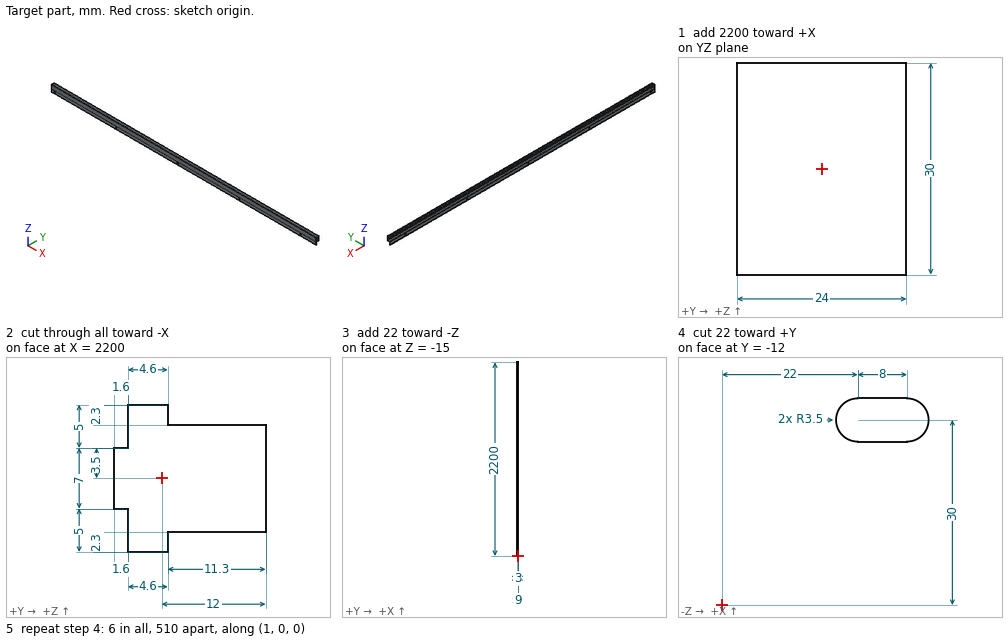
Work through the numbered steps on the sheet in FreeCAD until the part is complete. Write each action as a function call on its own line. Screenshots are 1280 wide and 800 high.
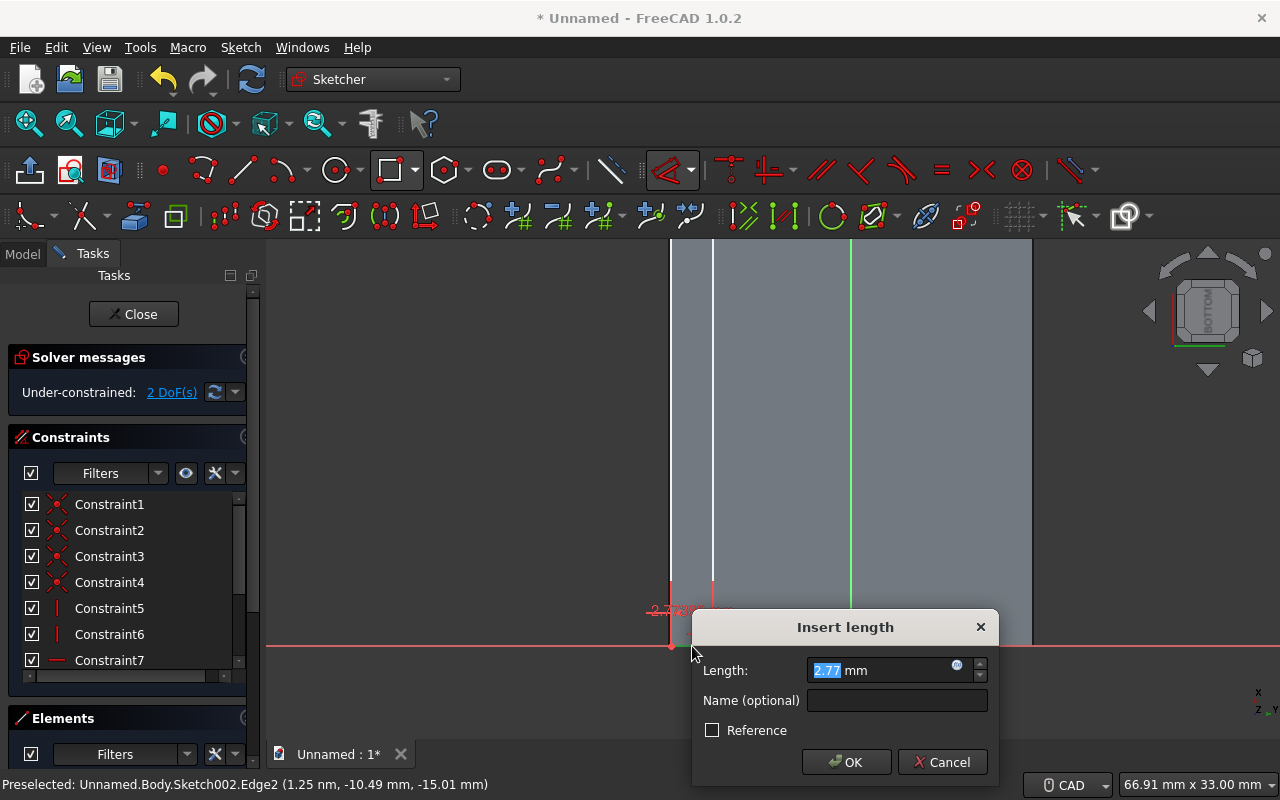
text(3)
key(Return)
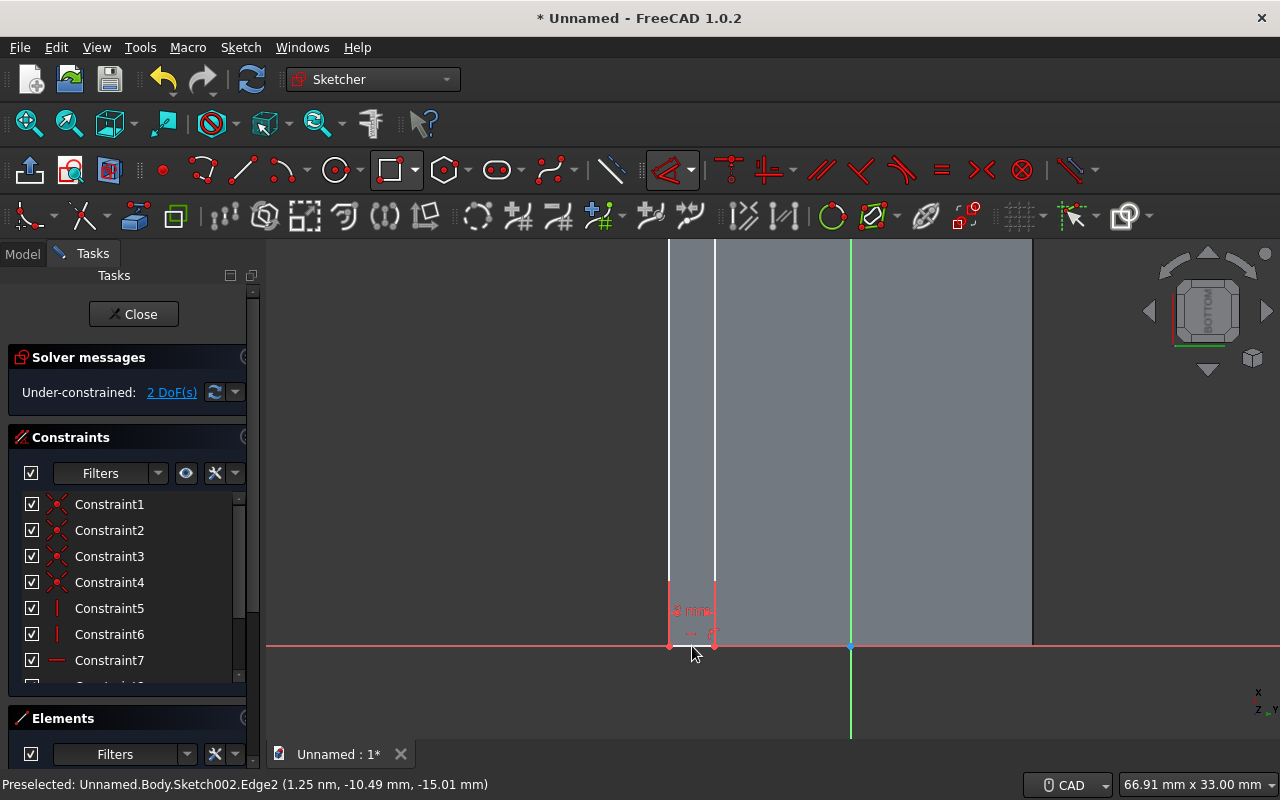
scroll(704, 489, down, 15)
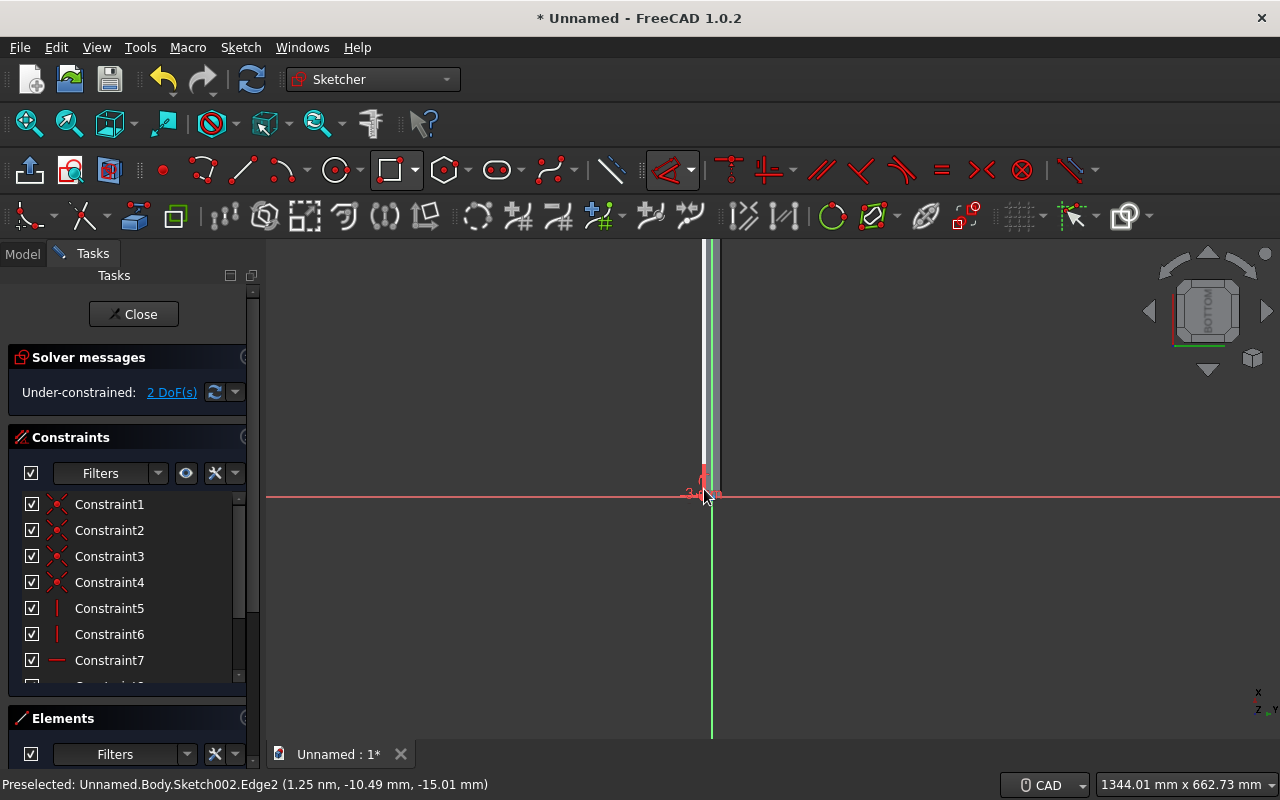
scroll(704, 697, down, 8)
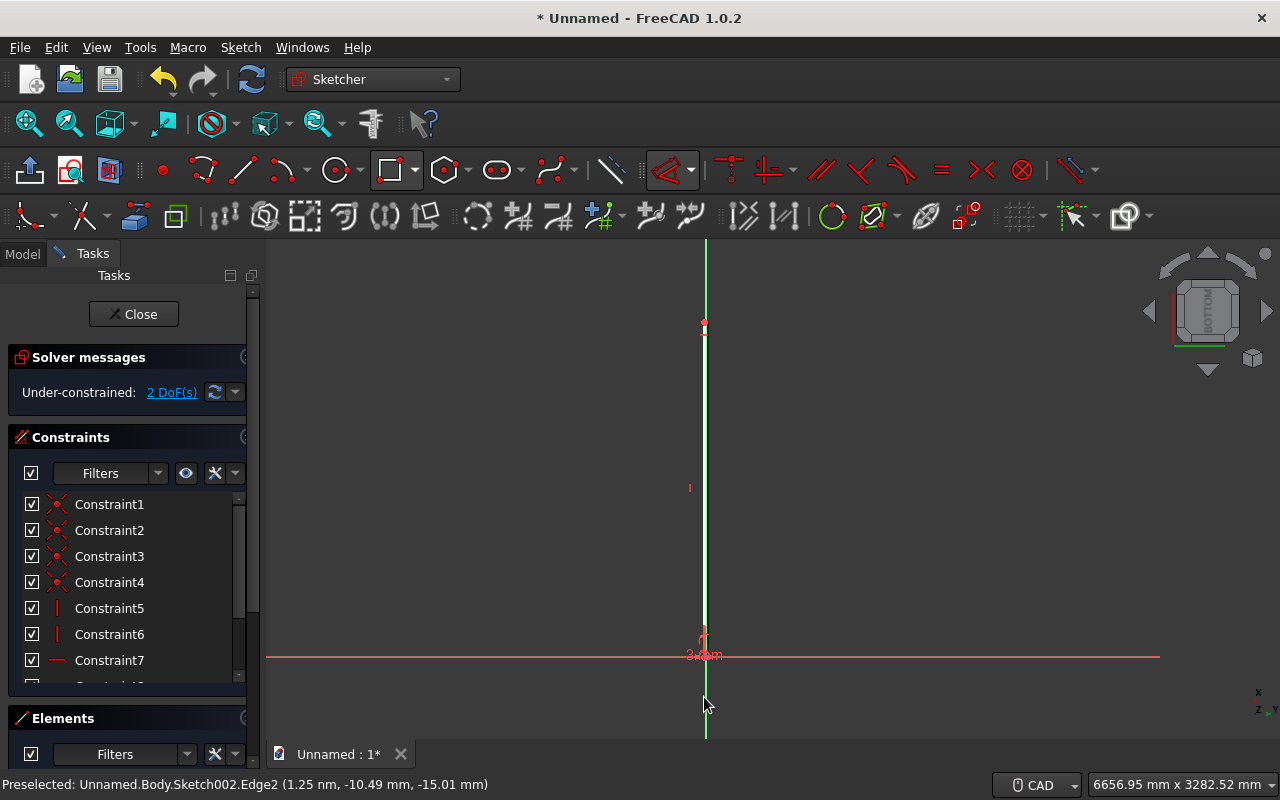
scroll(705, 657, up, 17)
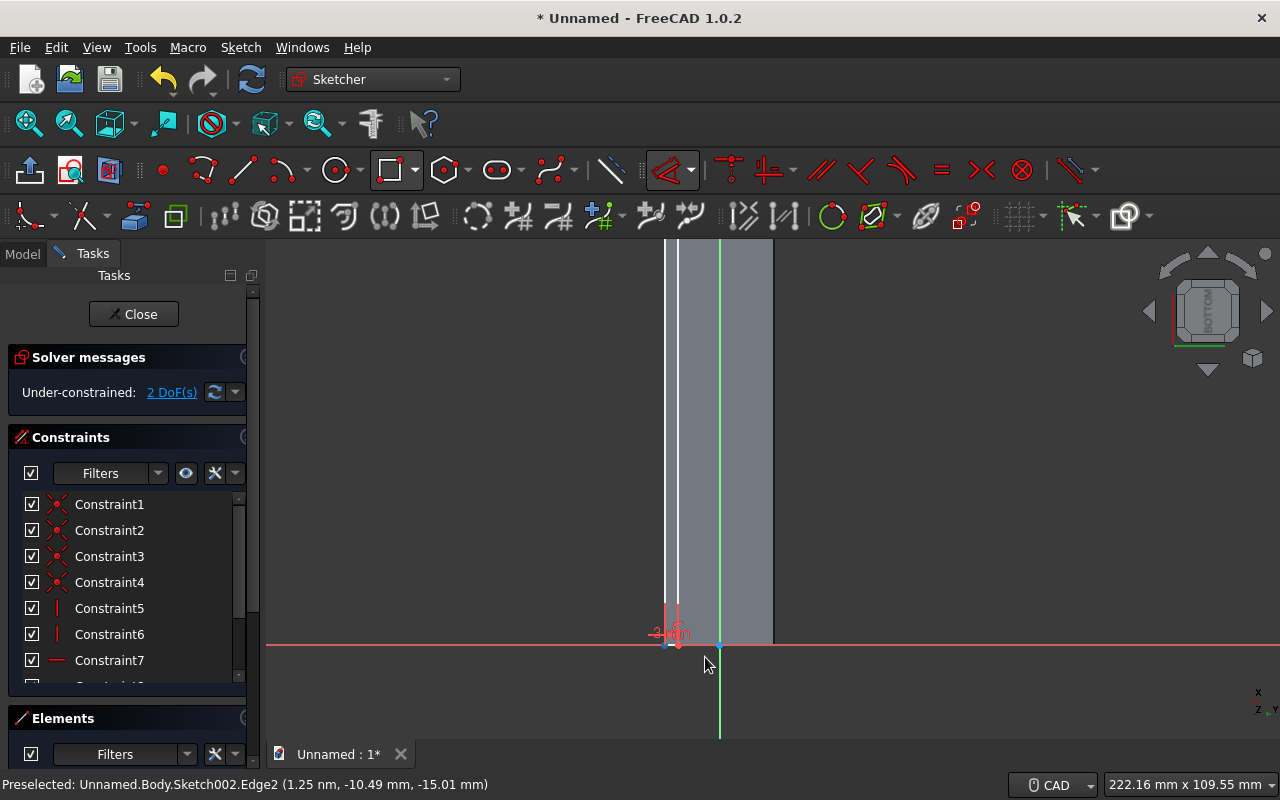
click(678, 645)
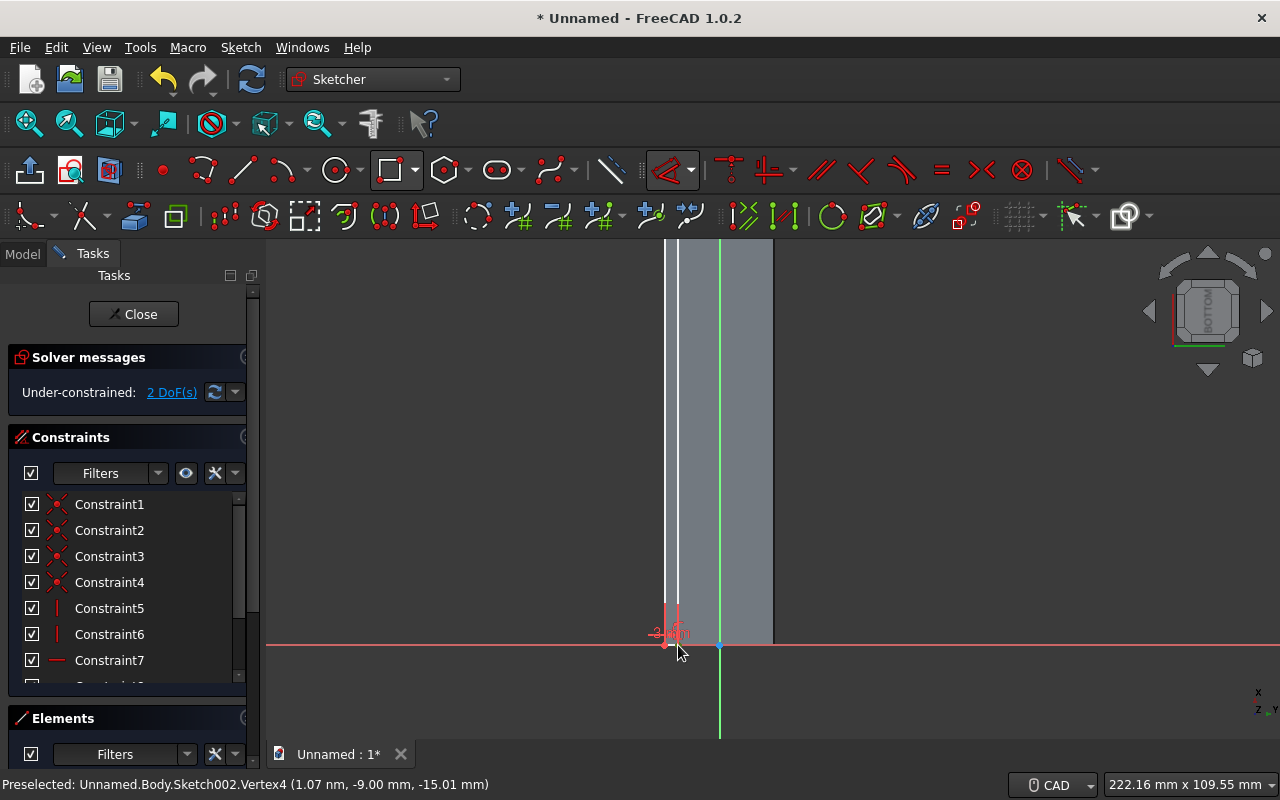
key(l)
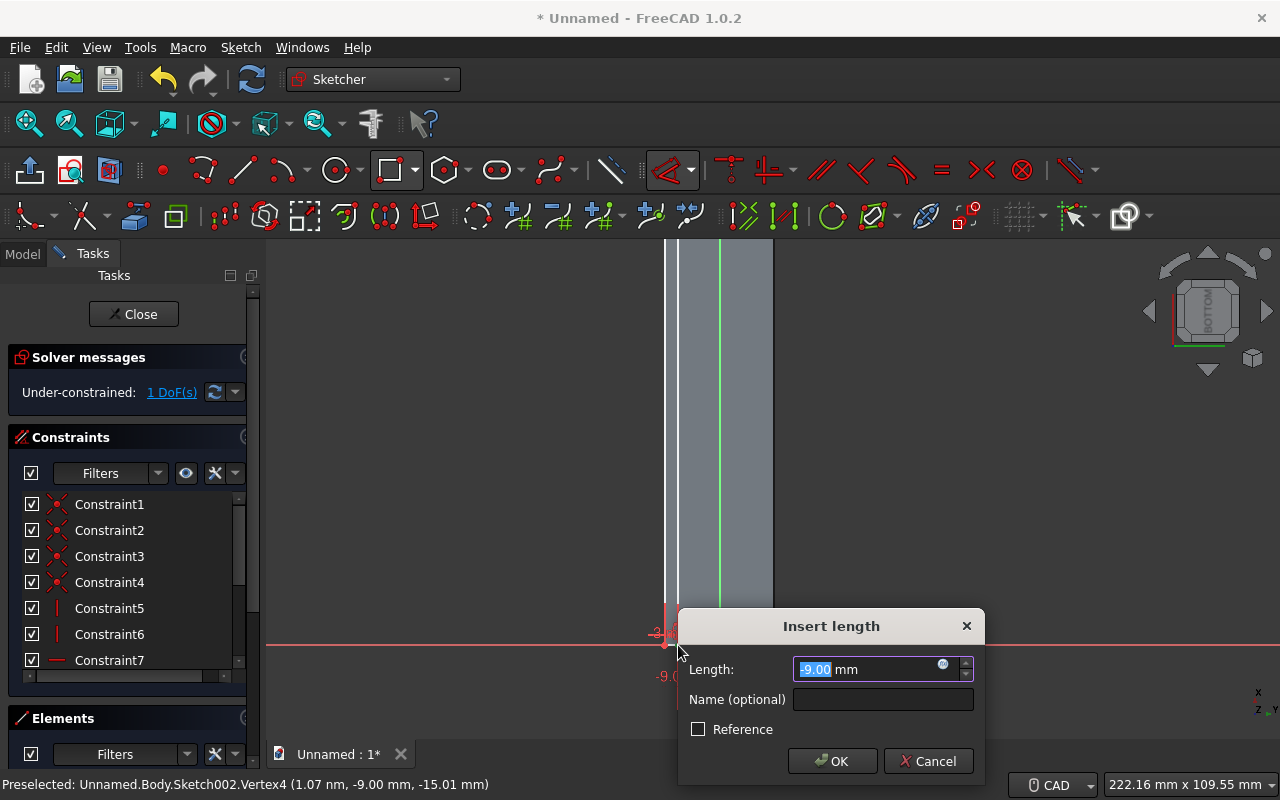
text(-9)
key(Return)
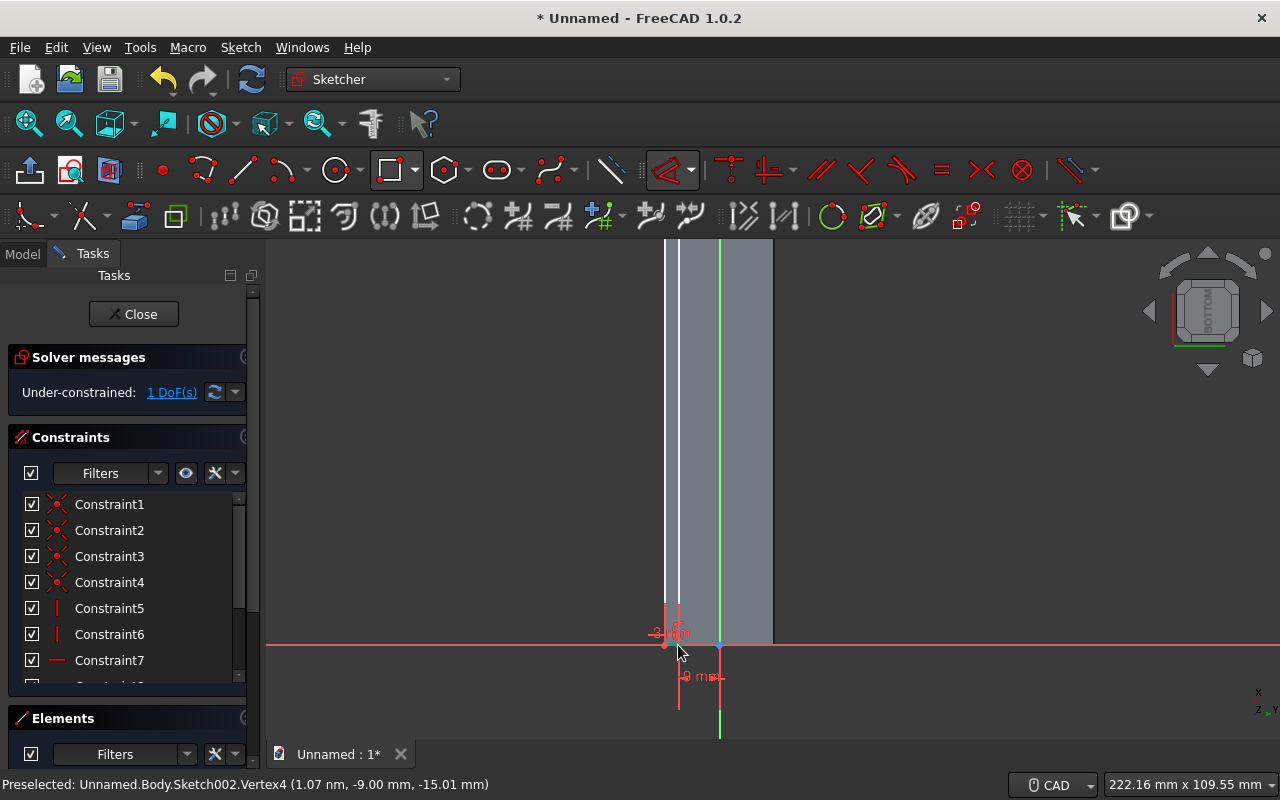
scroll(705, 657, down, 17)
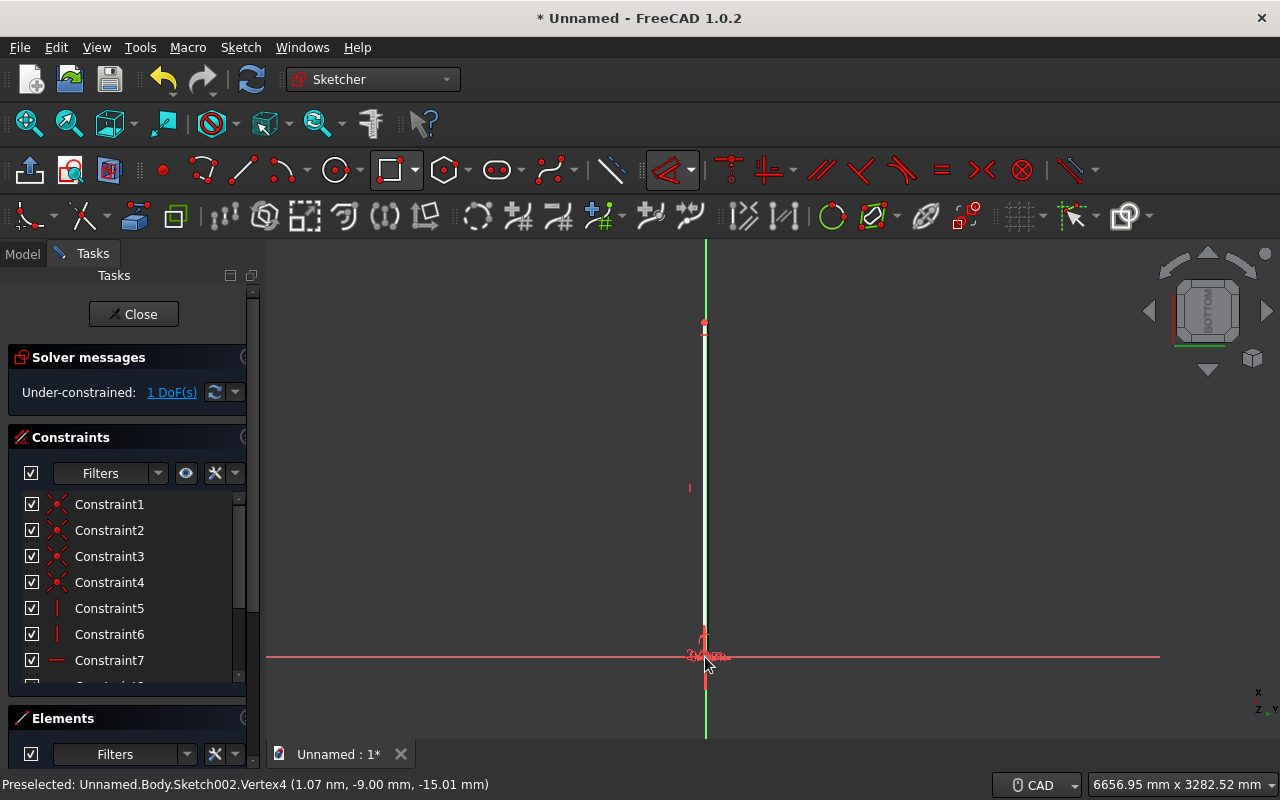
scroll(704, 423, up, 14)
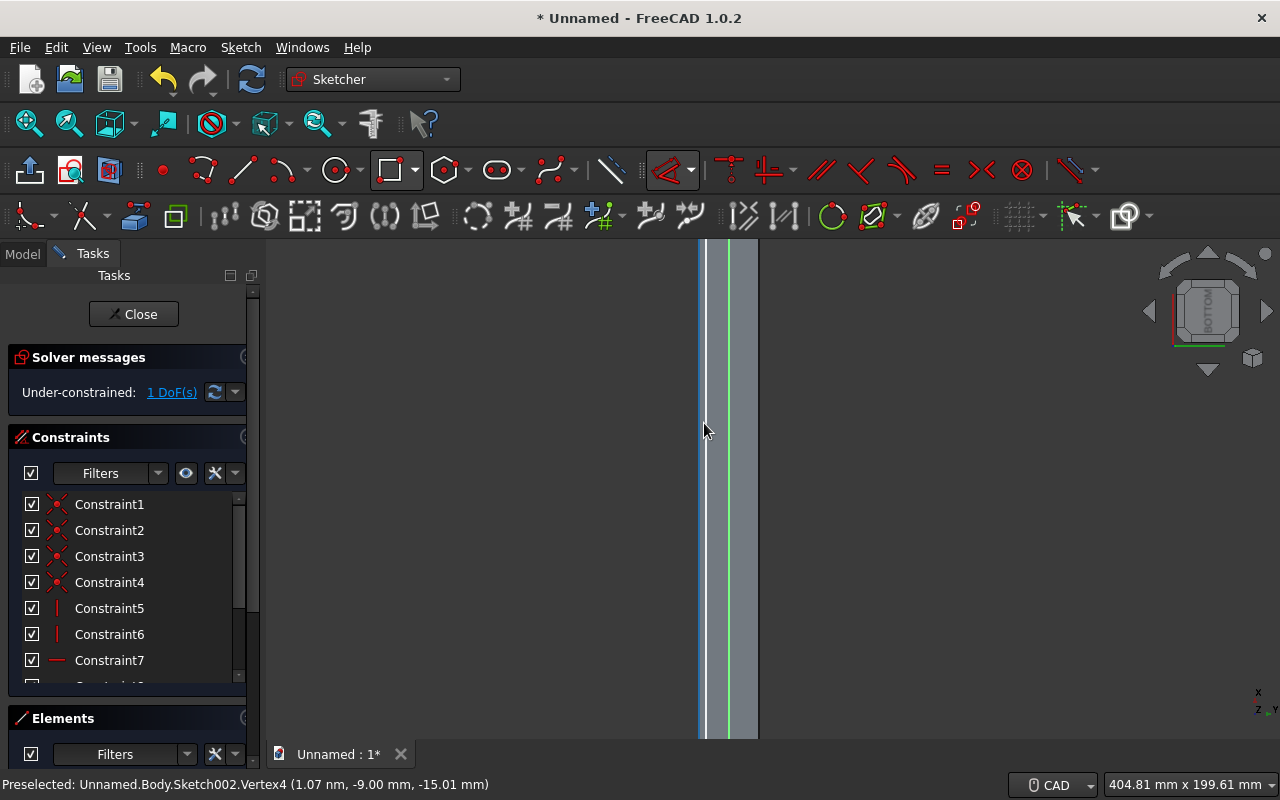
click(699, 416)